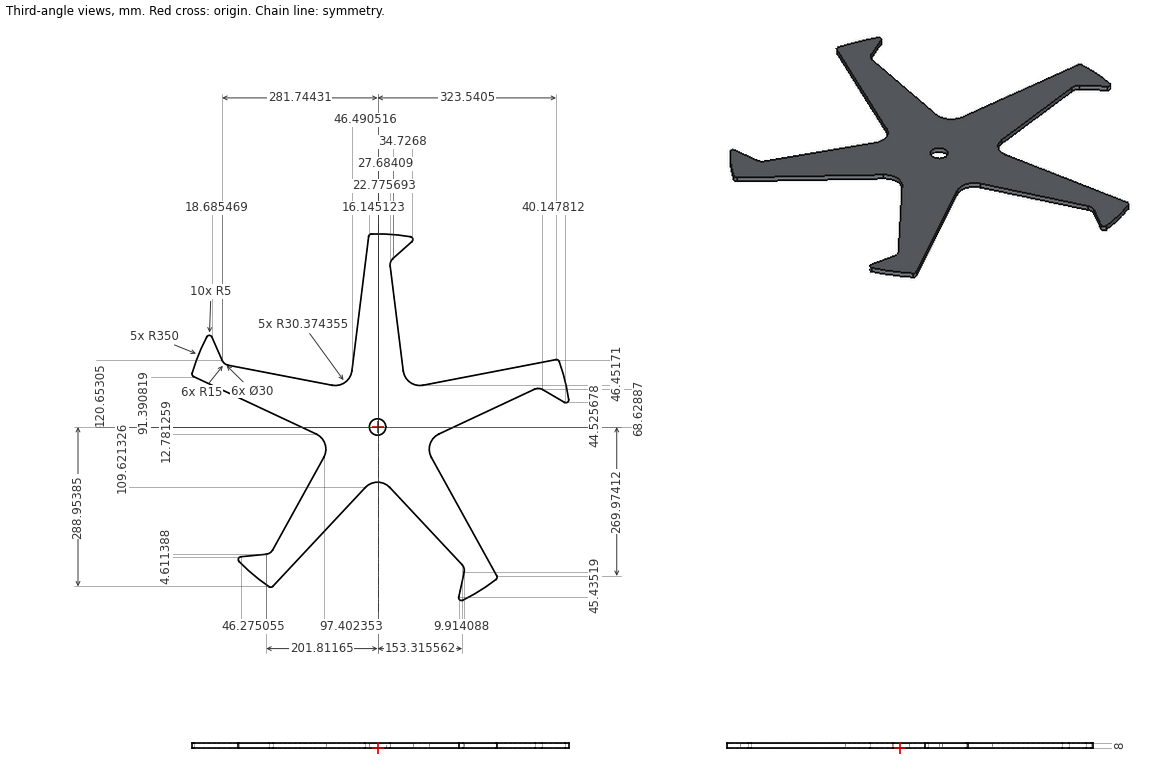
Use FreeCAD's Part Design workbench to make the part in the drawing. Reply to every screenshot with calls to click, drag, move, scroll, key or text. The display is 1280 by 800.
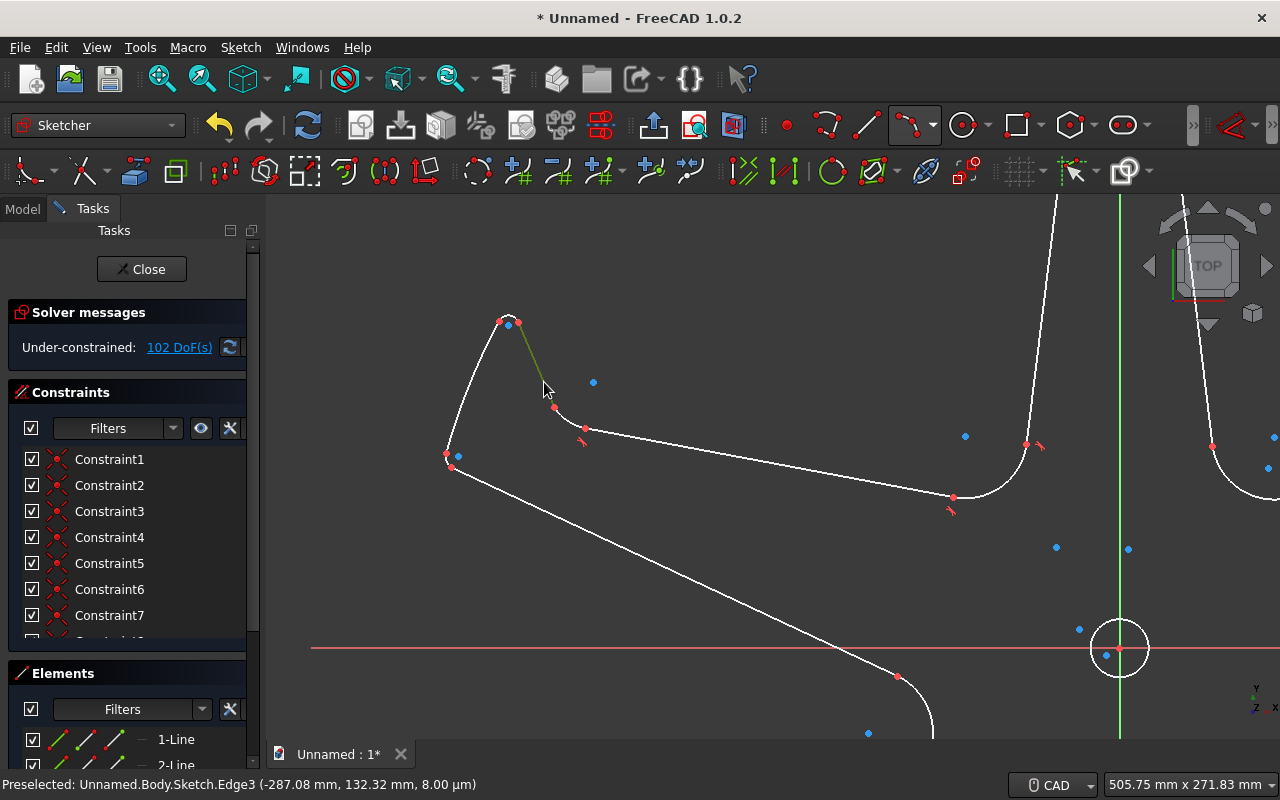
click(562, 416)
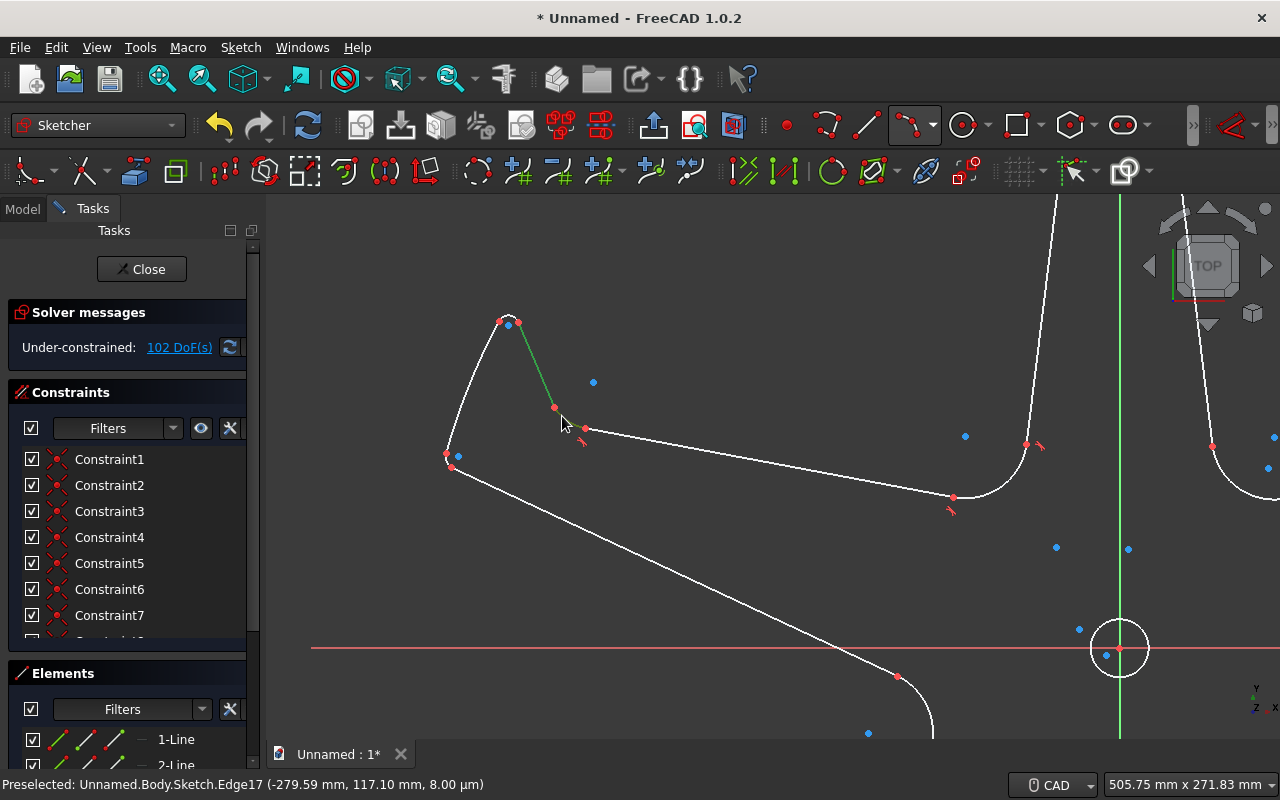
key(t)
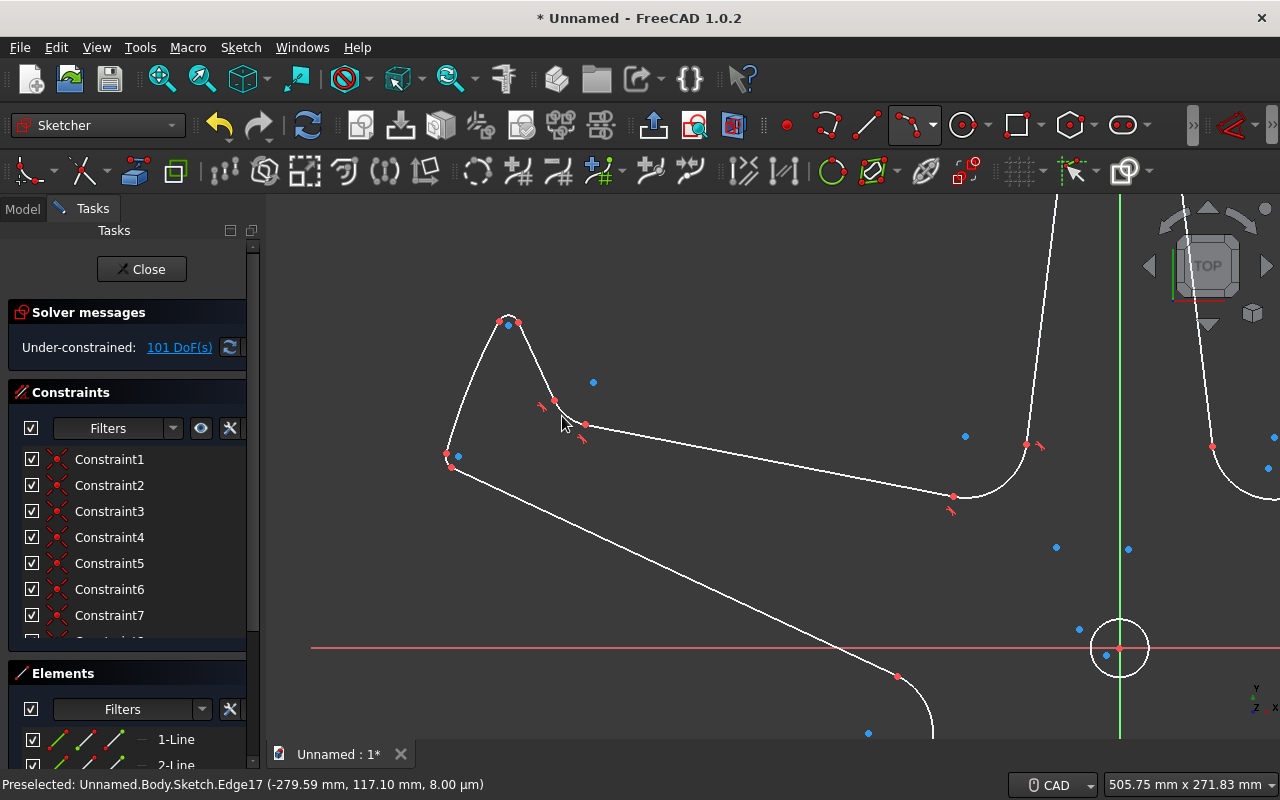
click(544, 377)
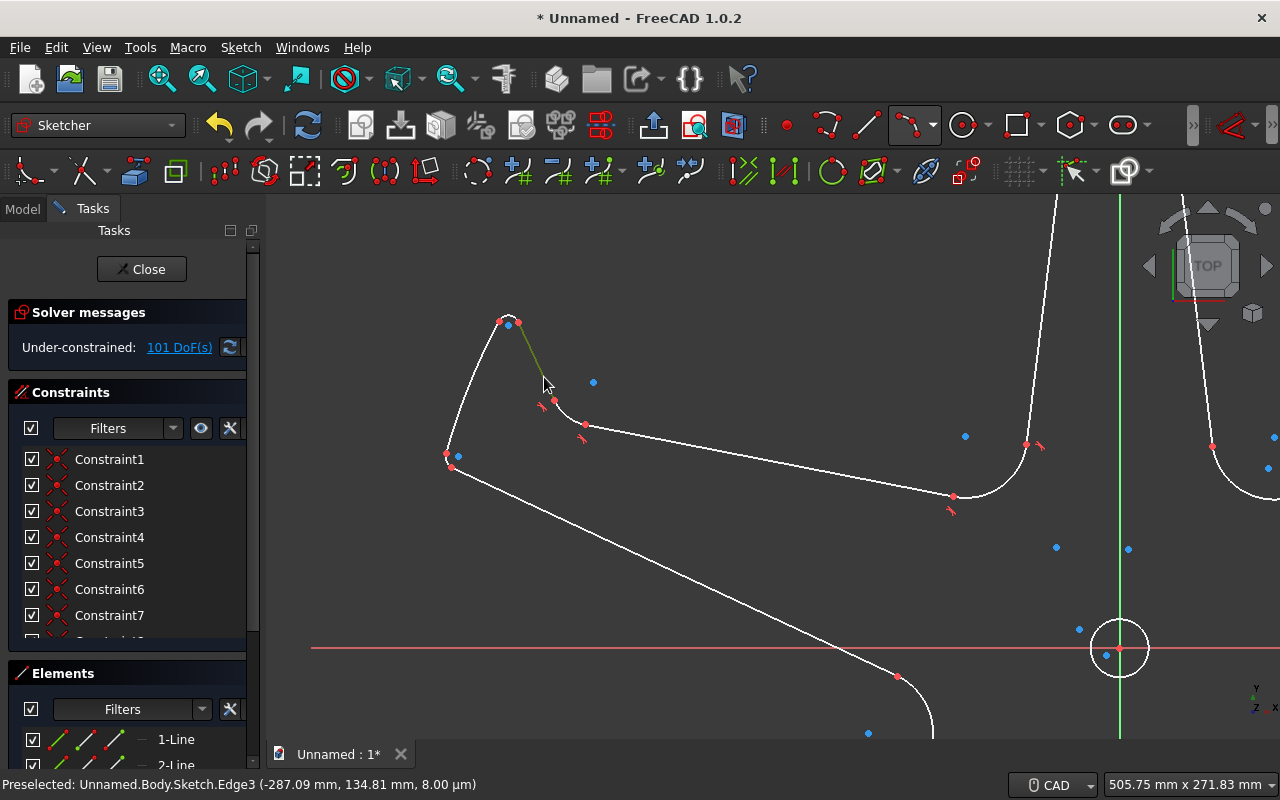
scroll(509, 315, up, 2)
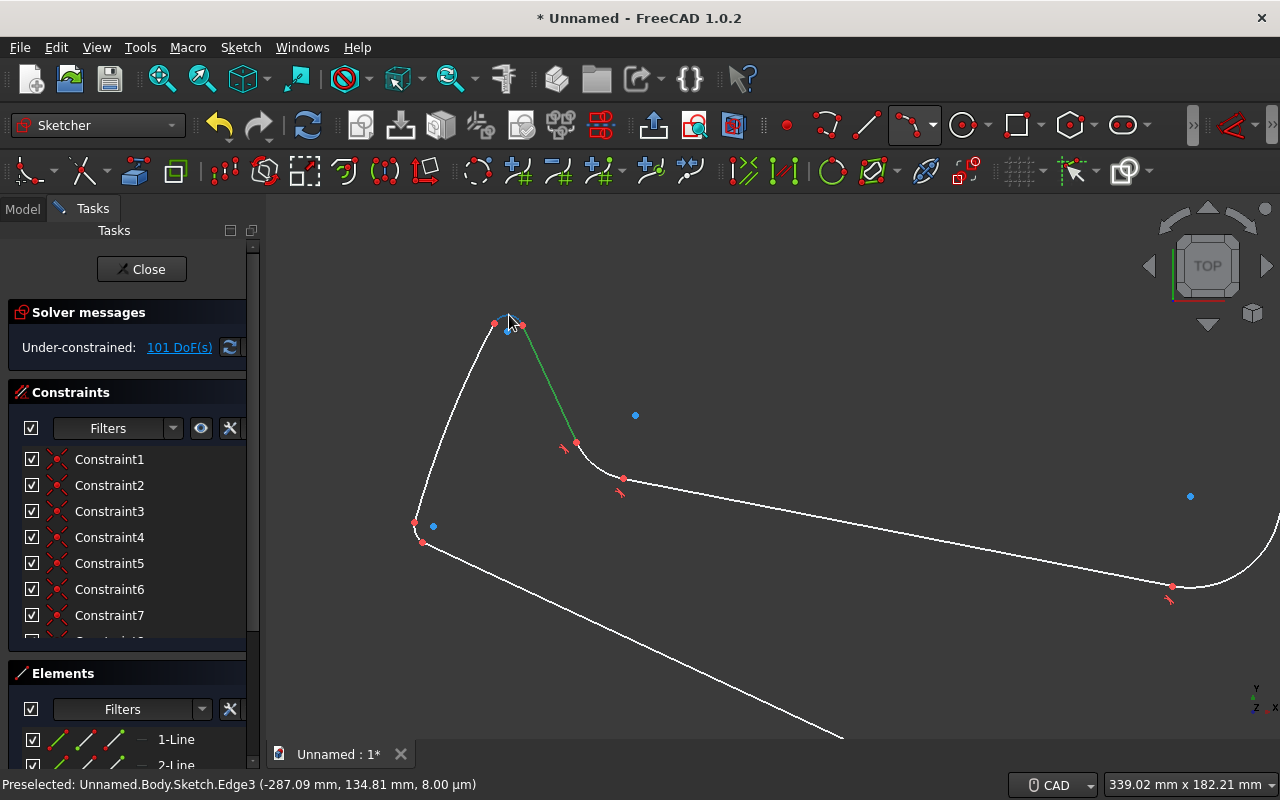
click(509, 315)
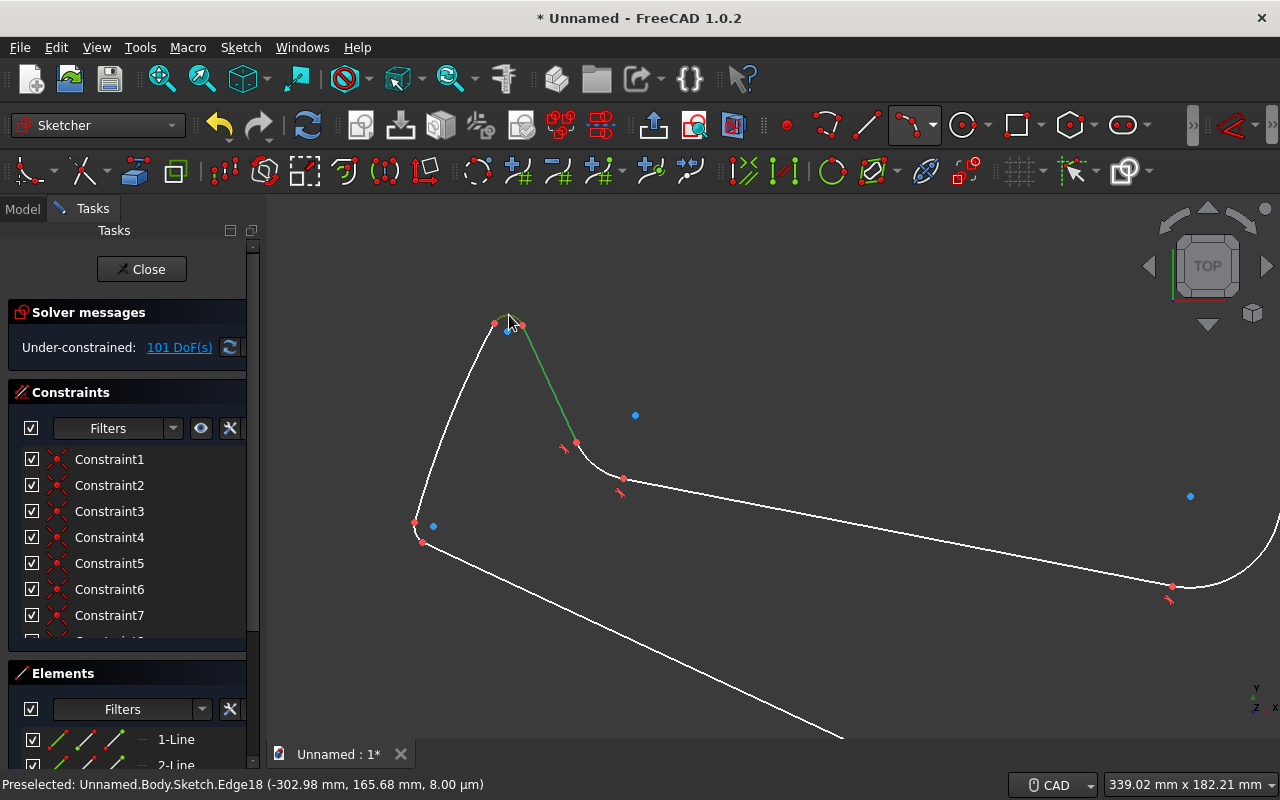
key(t)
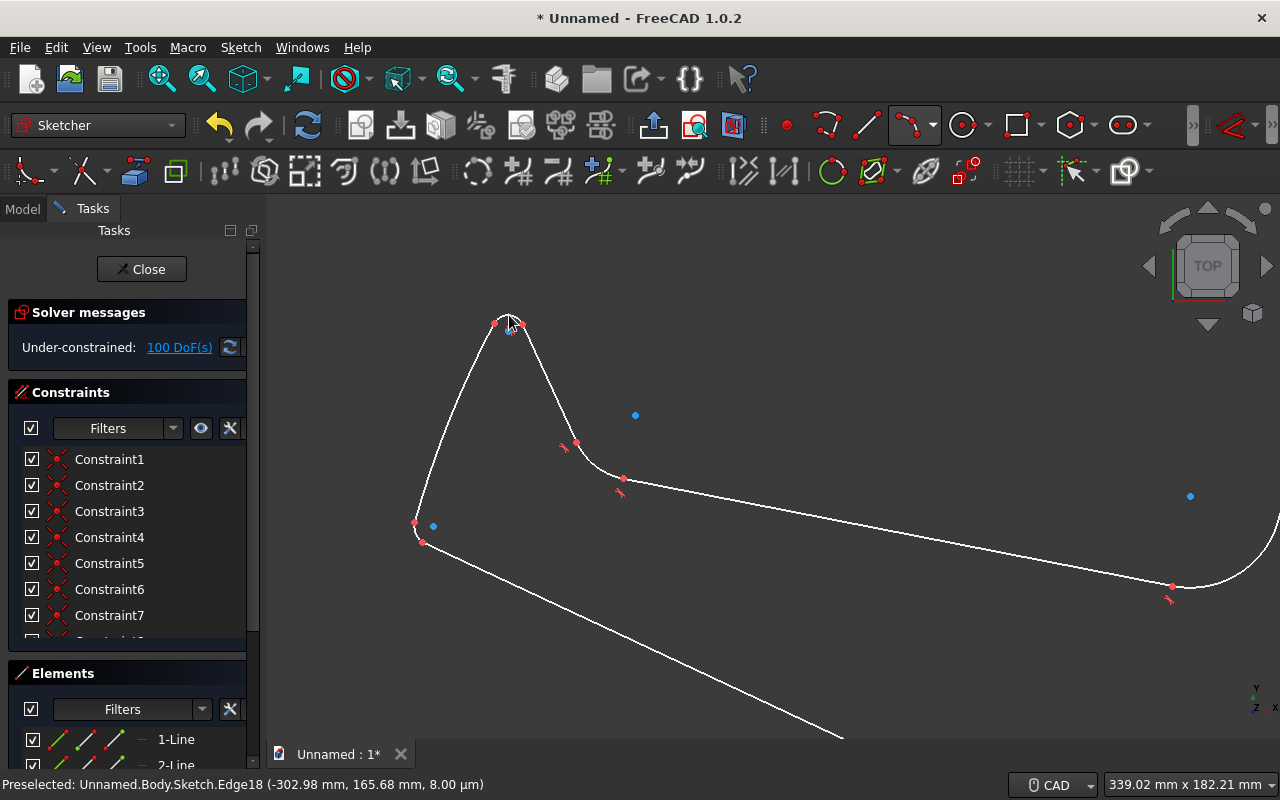
scroll(560, 409, down, 9)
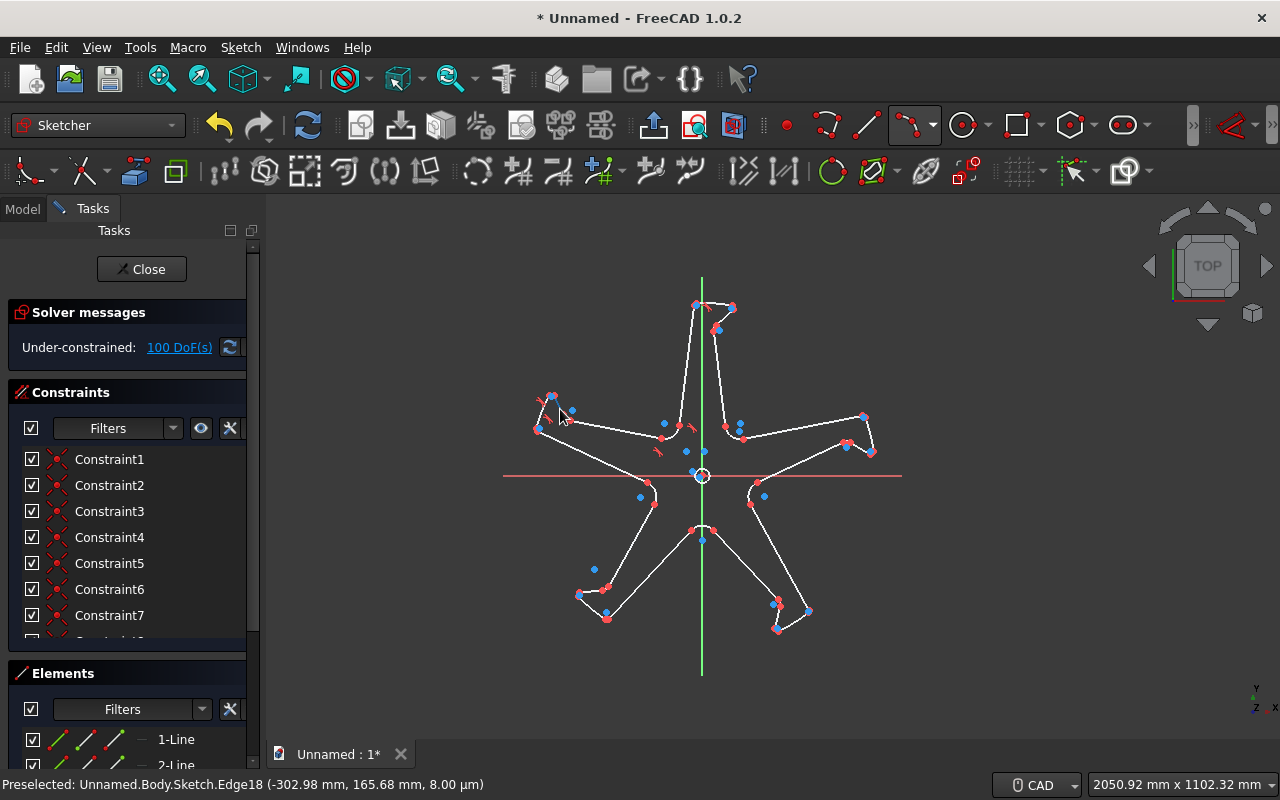
click(571, 447)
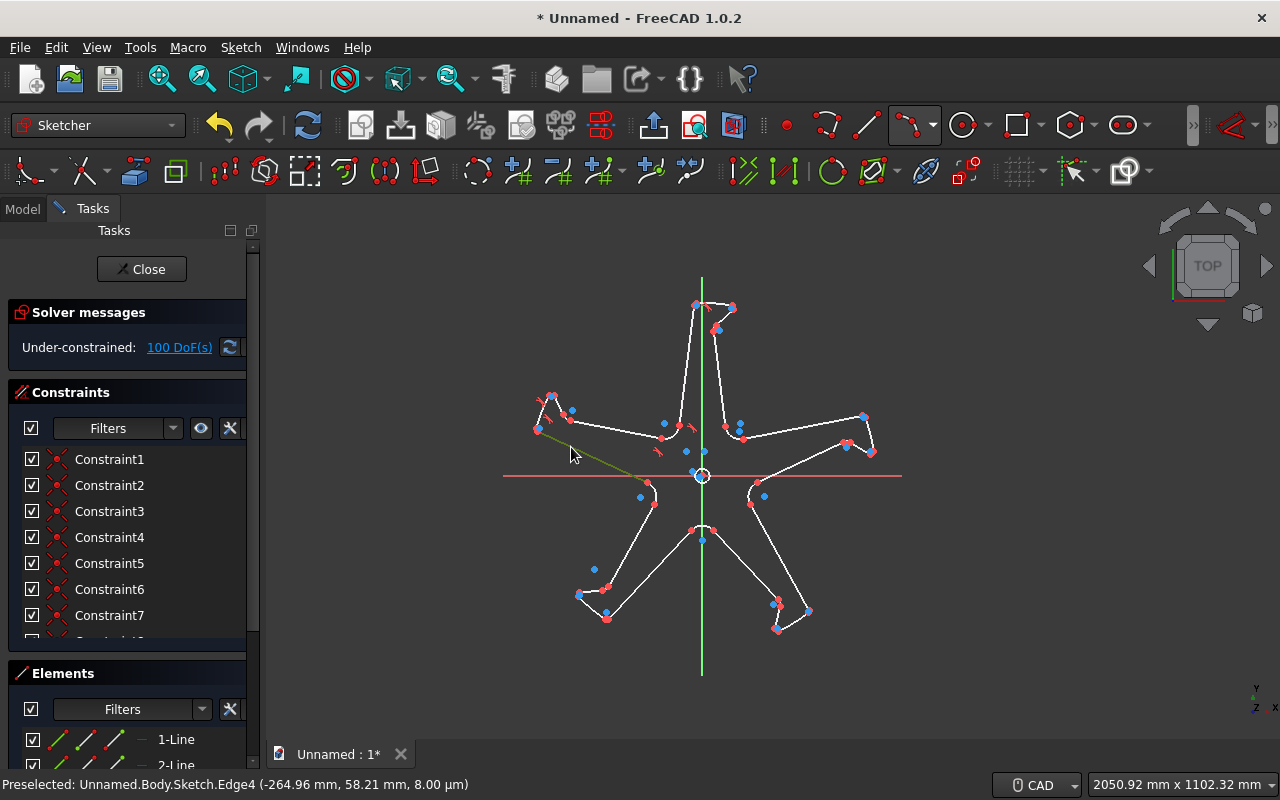
scroll(536, 430, up, 11)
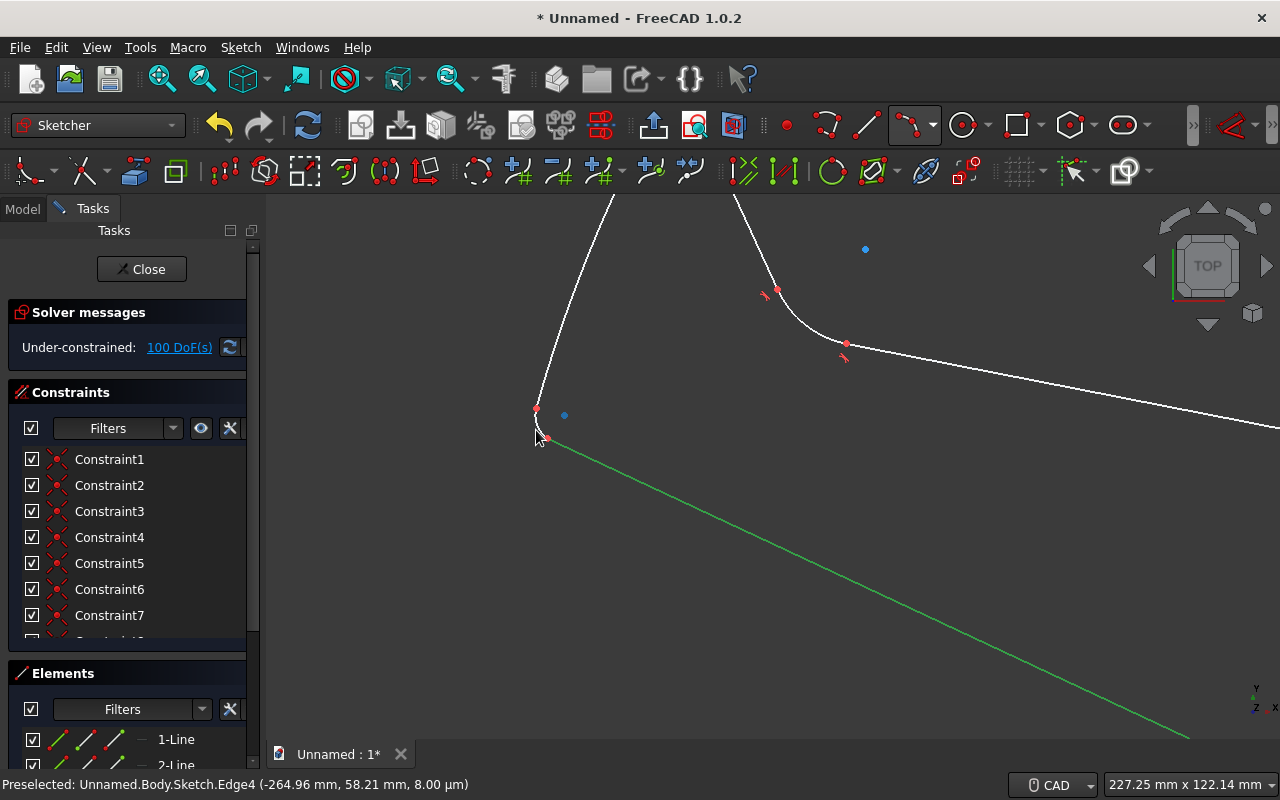
click(537, 425)